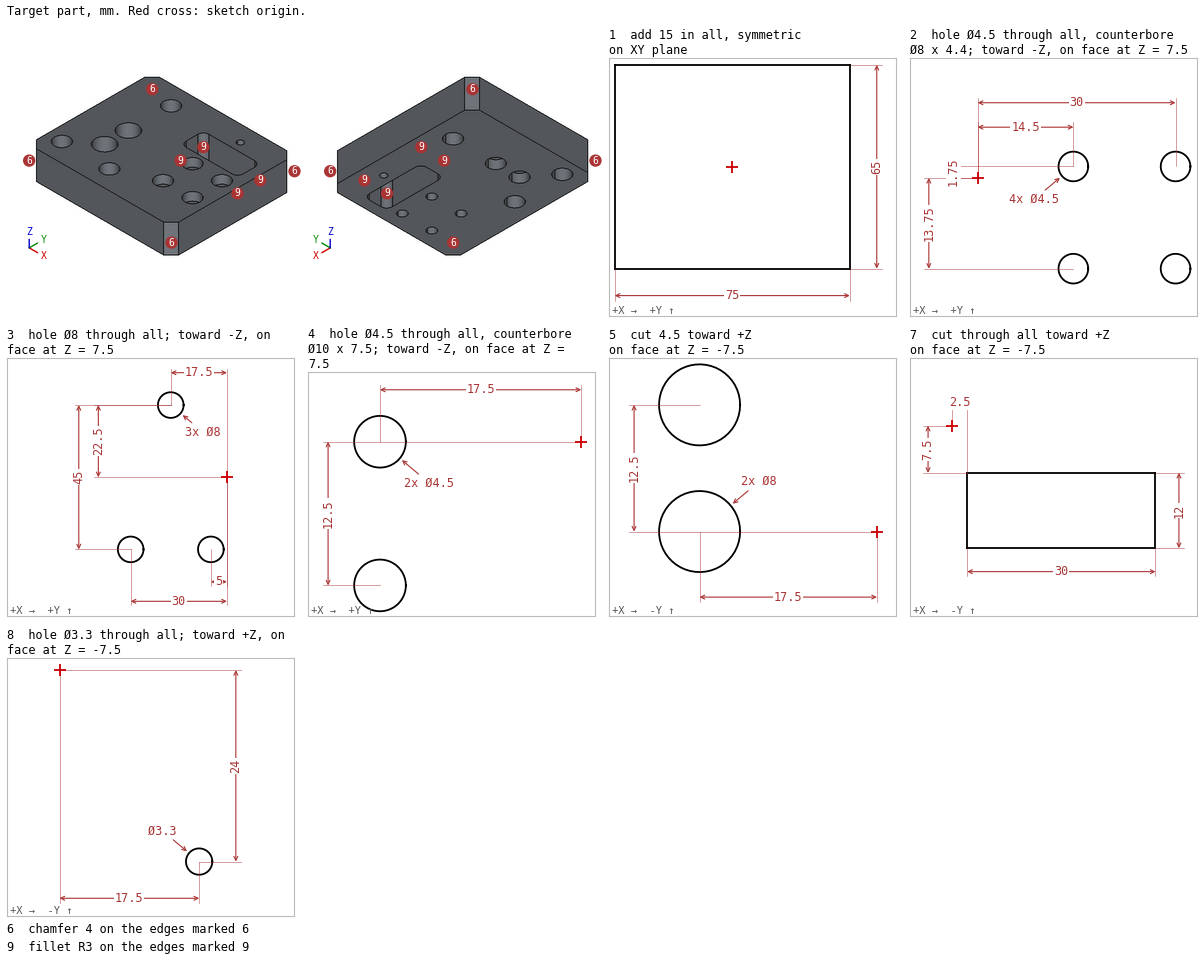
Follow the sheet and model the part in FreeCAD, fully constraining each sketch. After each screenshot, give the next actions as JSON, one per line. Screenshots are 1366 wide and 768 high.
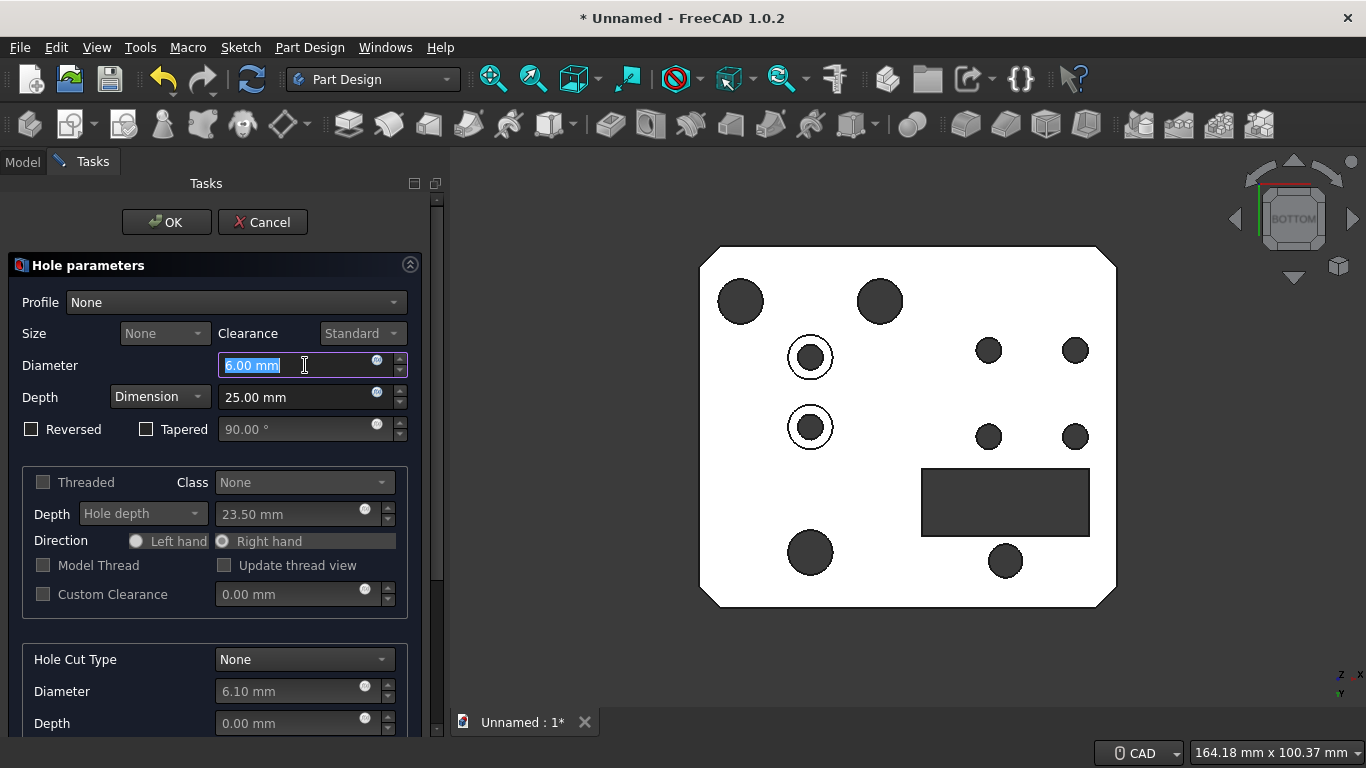
{"action": "type", "text": "3.3"}
{"action": "key", "text": "Tab"}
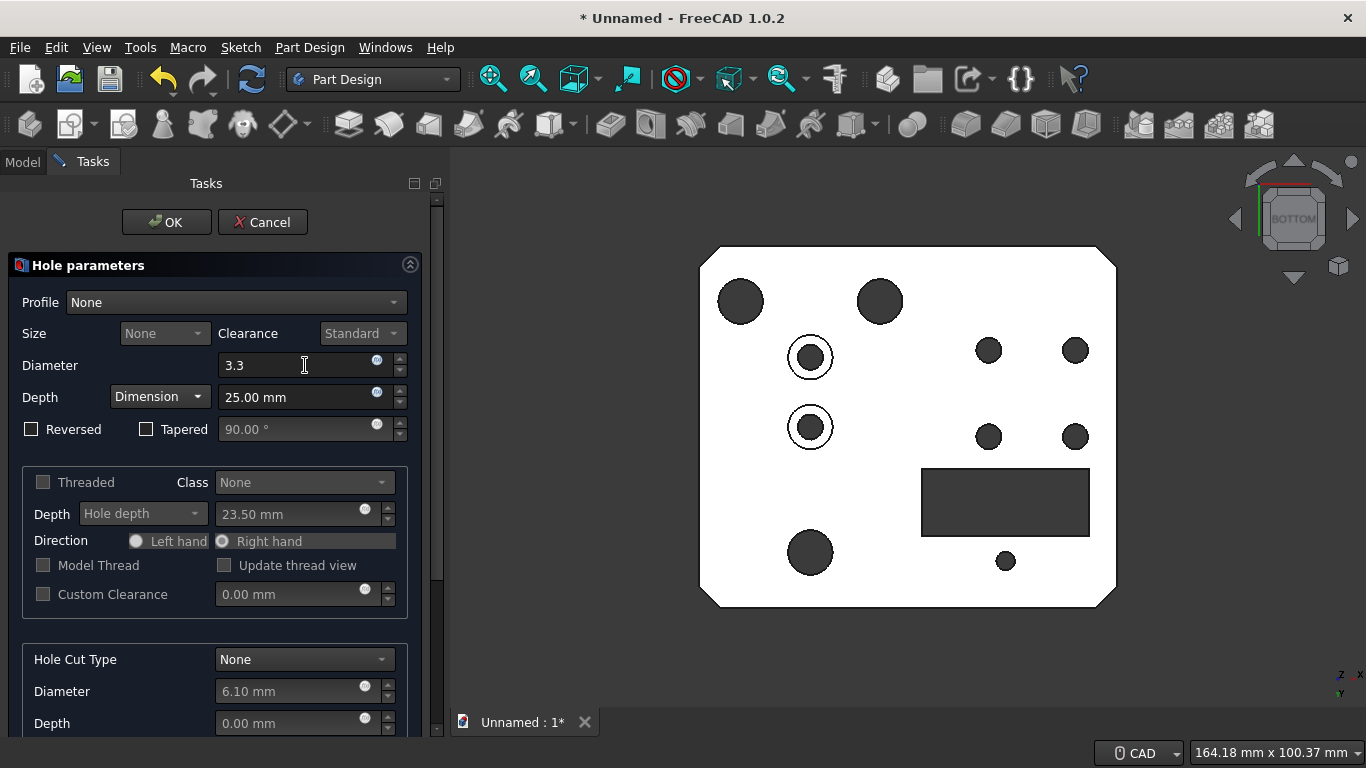
{"action": "left_click", "coordinate": [161, 396]}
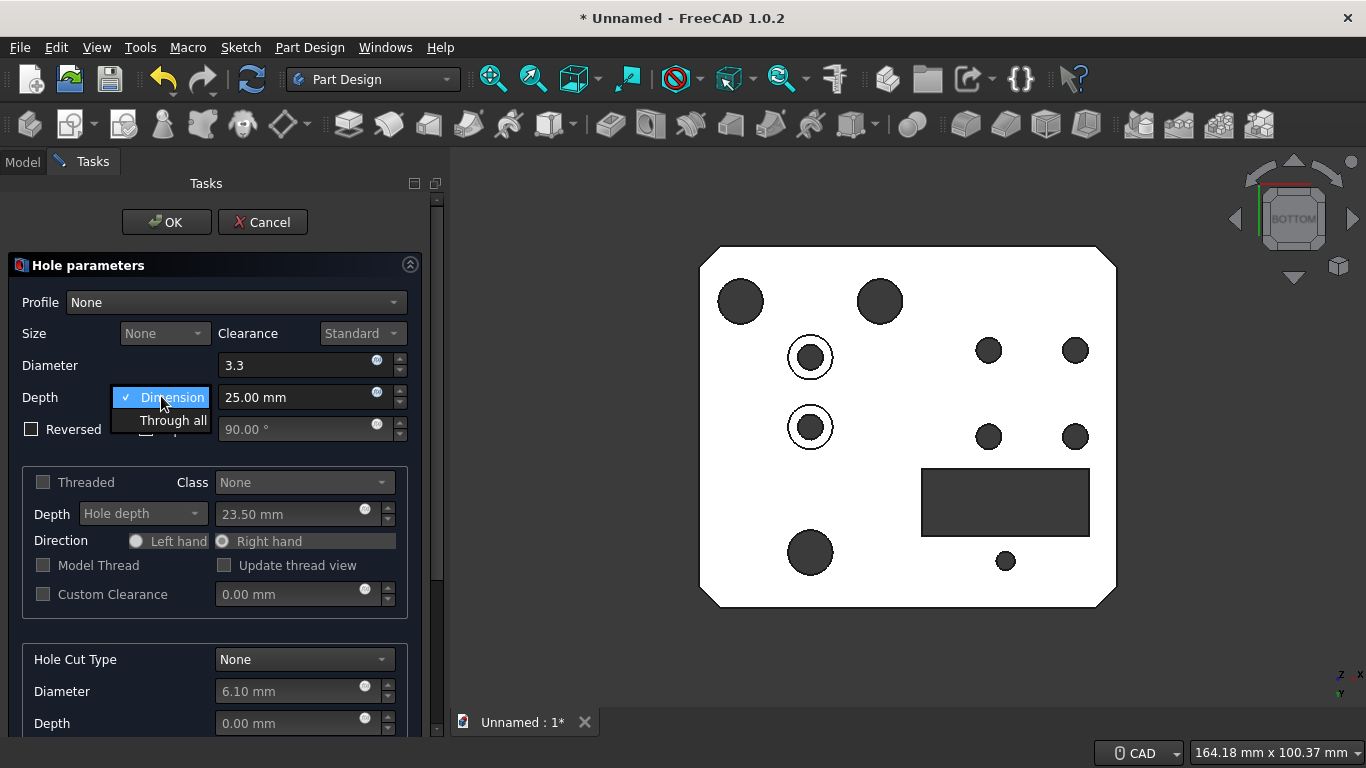
{"action": "left_click", "coordinate": [160, 420]}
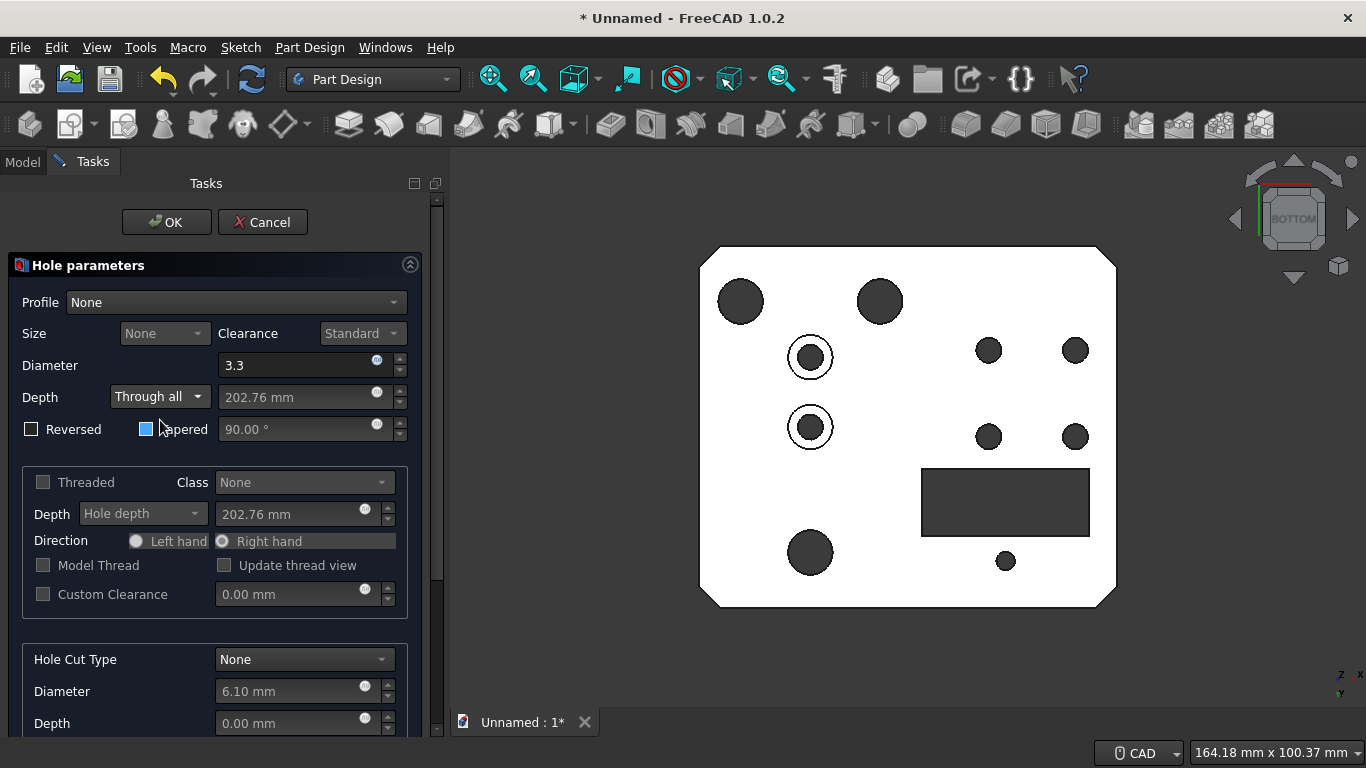
{"action": "left_click", "coordinate": [167, 222]}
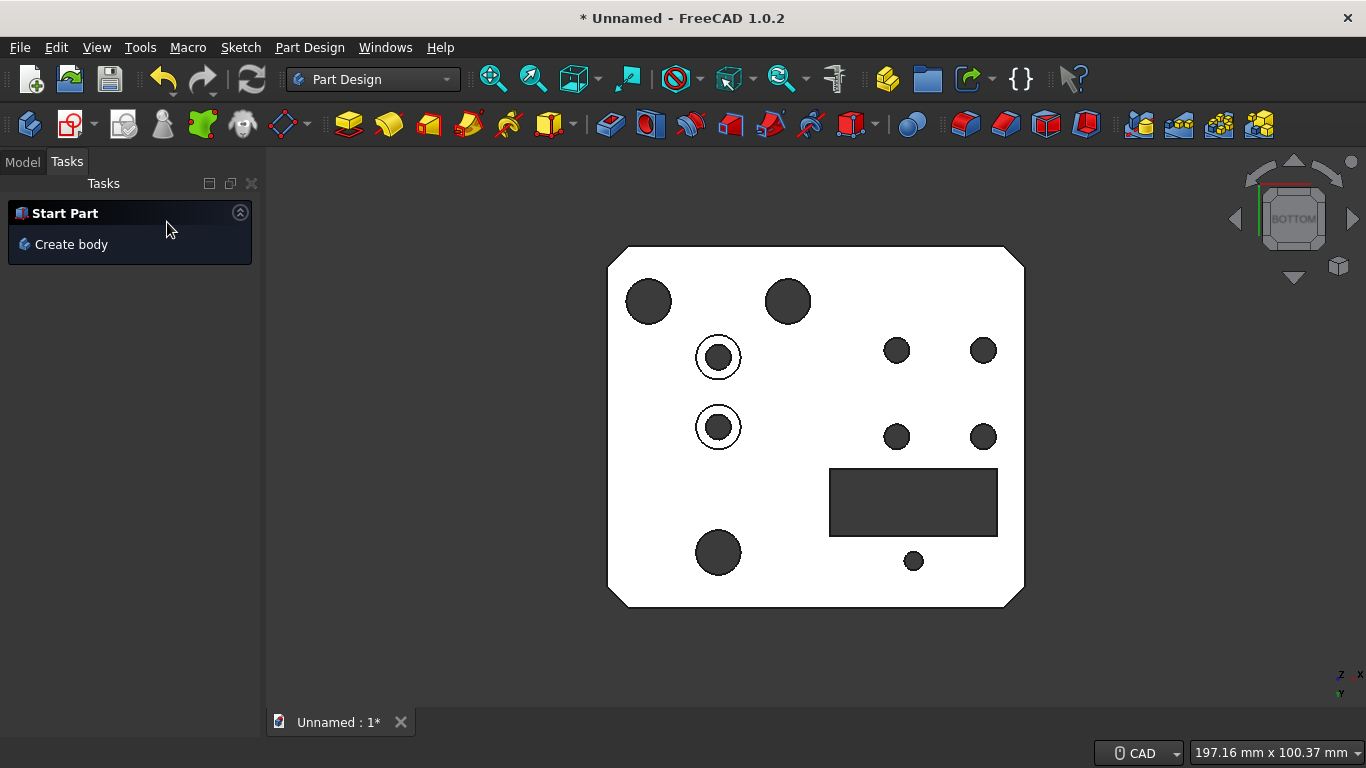
{"action": "key", "text": "0"}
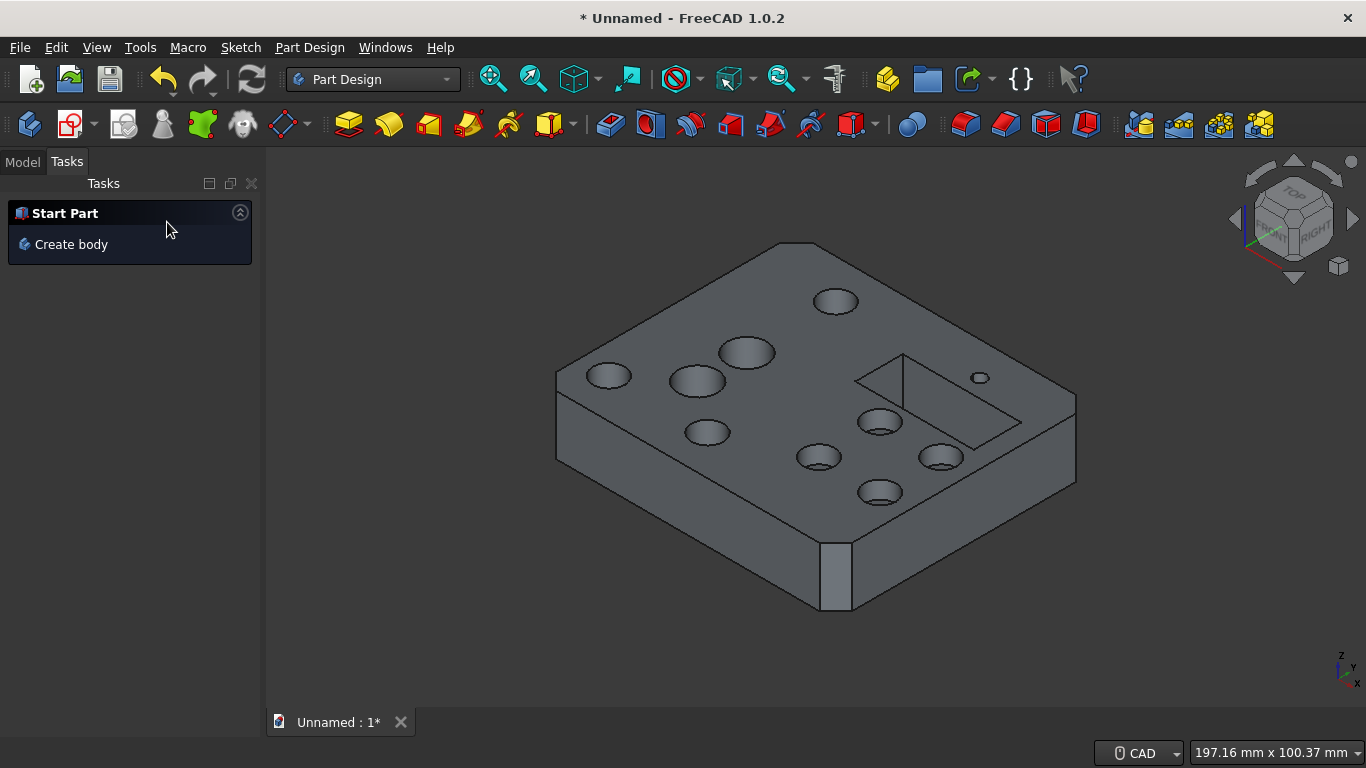
{"action": "key", "text": "2"}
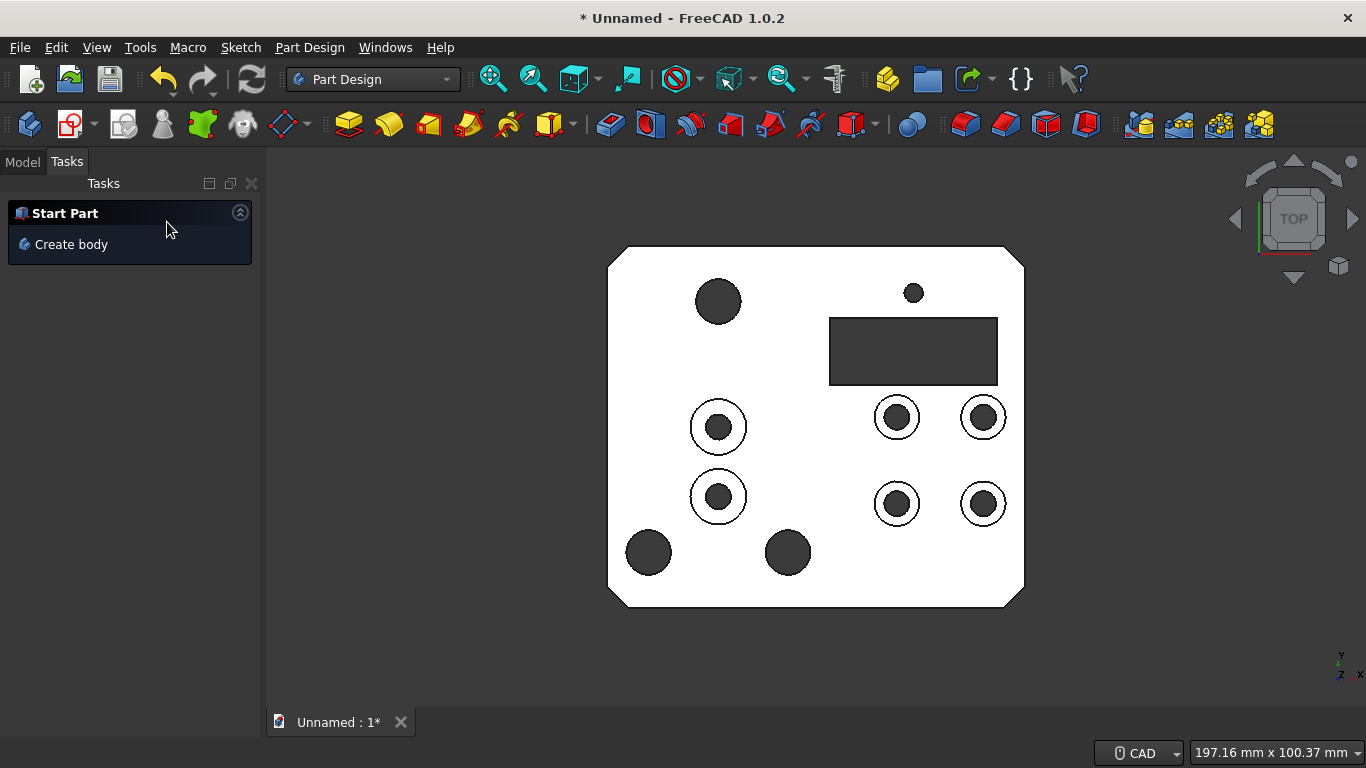
{"action": "key", "text": "1"}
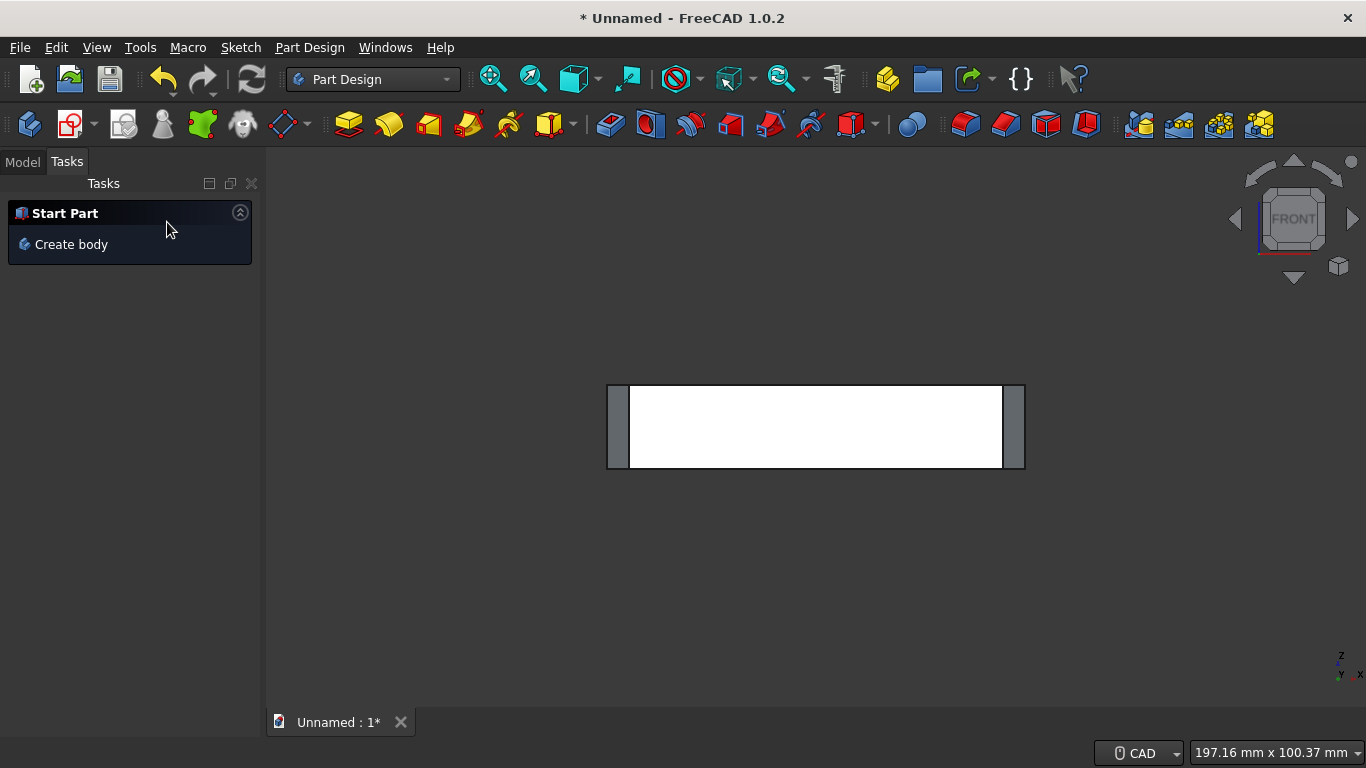
{"action": "key", "text": "v f"}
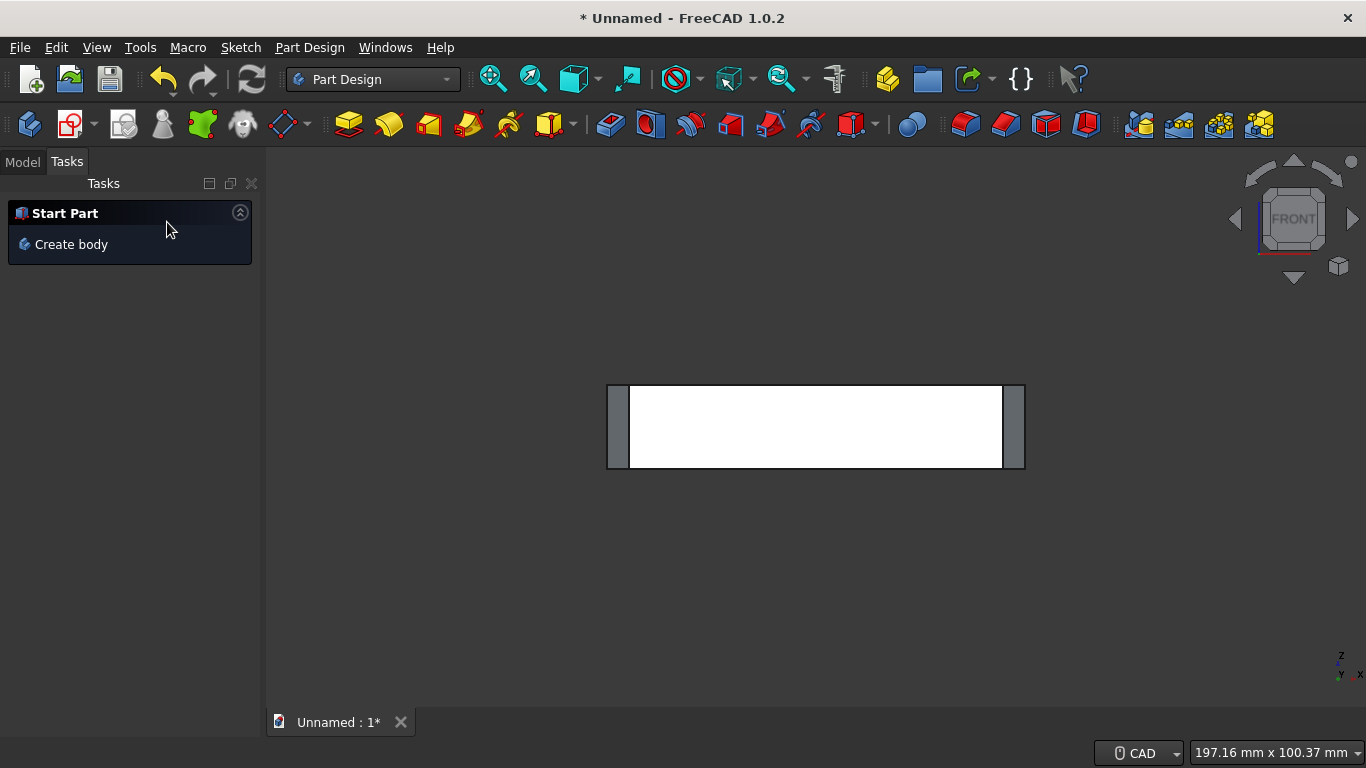
{"action": "key", "text": "3"}